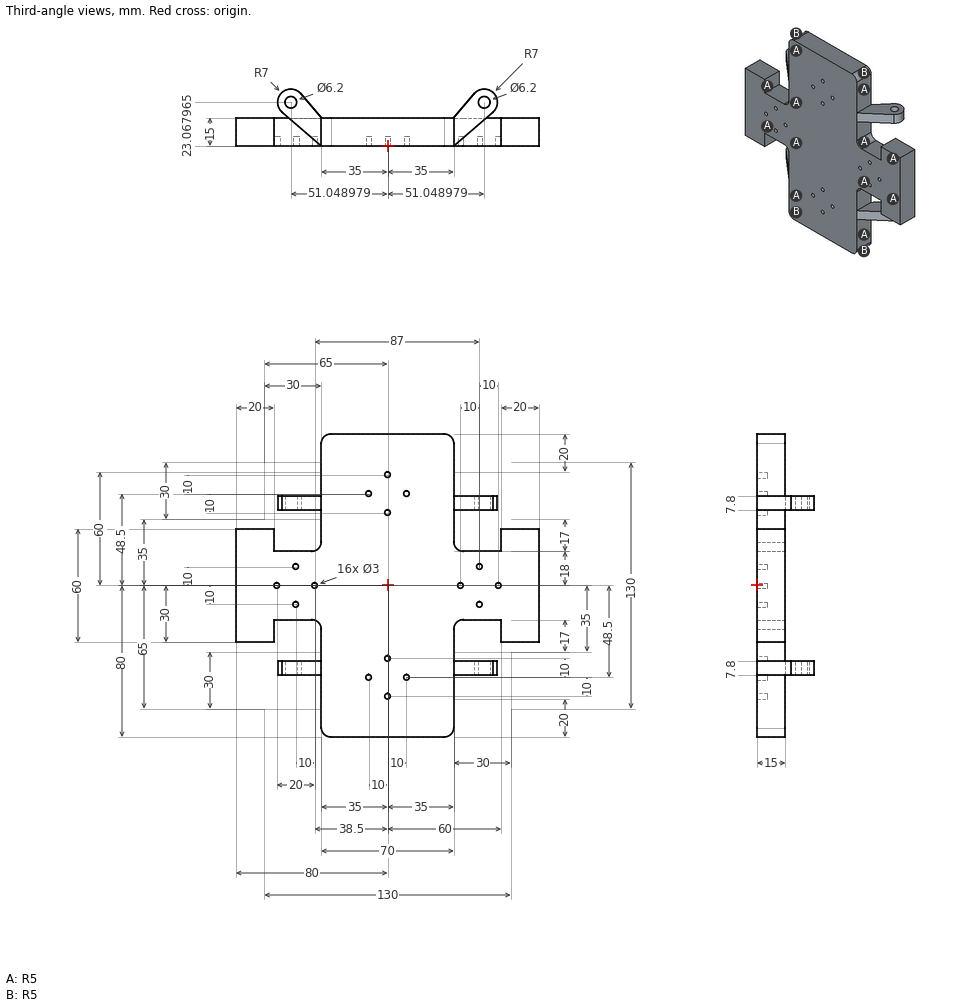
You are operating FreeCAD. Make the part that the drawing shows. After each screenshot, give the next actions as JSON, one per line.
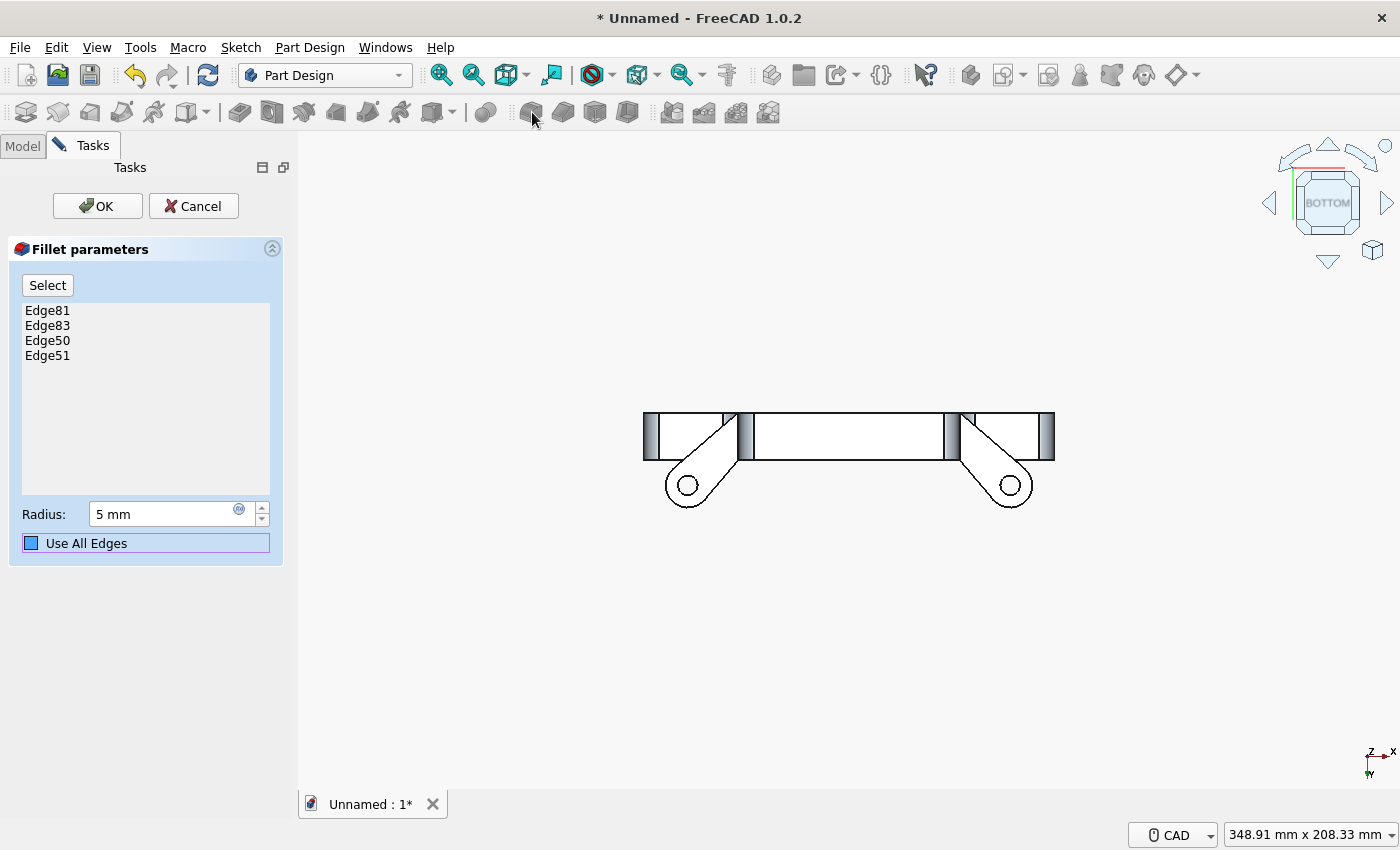
{"action": "left_click", "coordinate": [98, 206]}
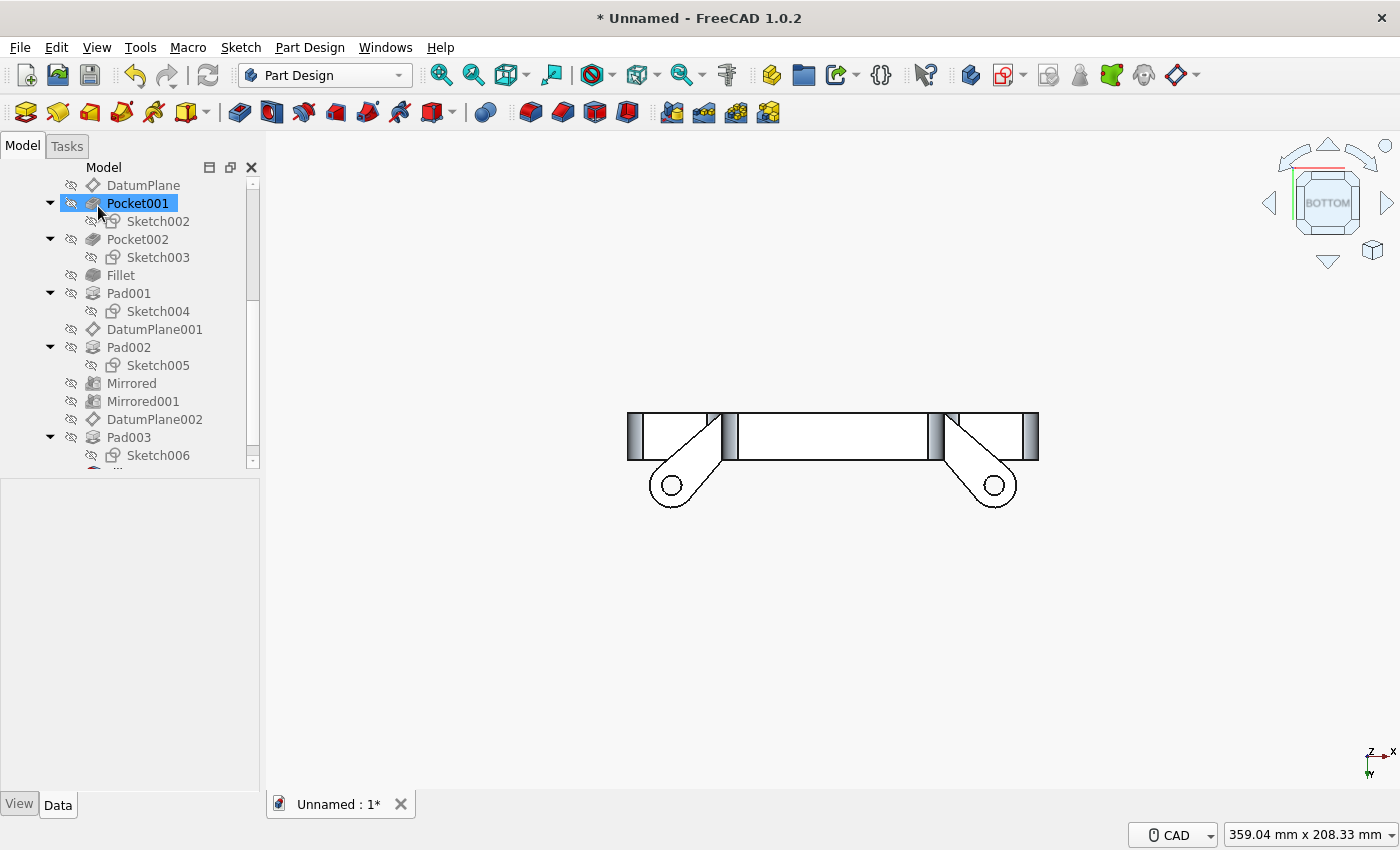
{"action": "left_click", "coordinate": [442, 76]}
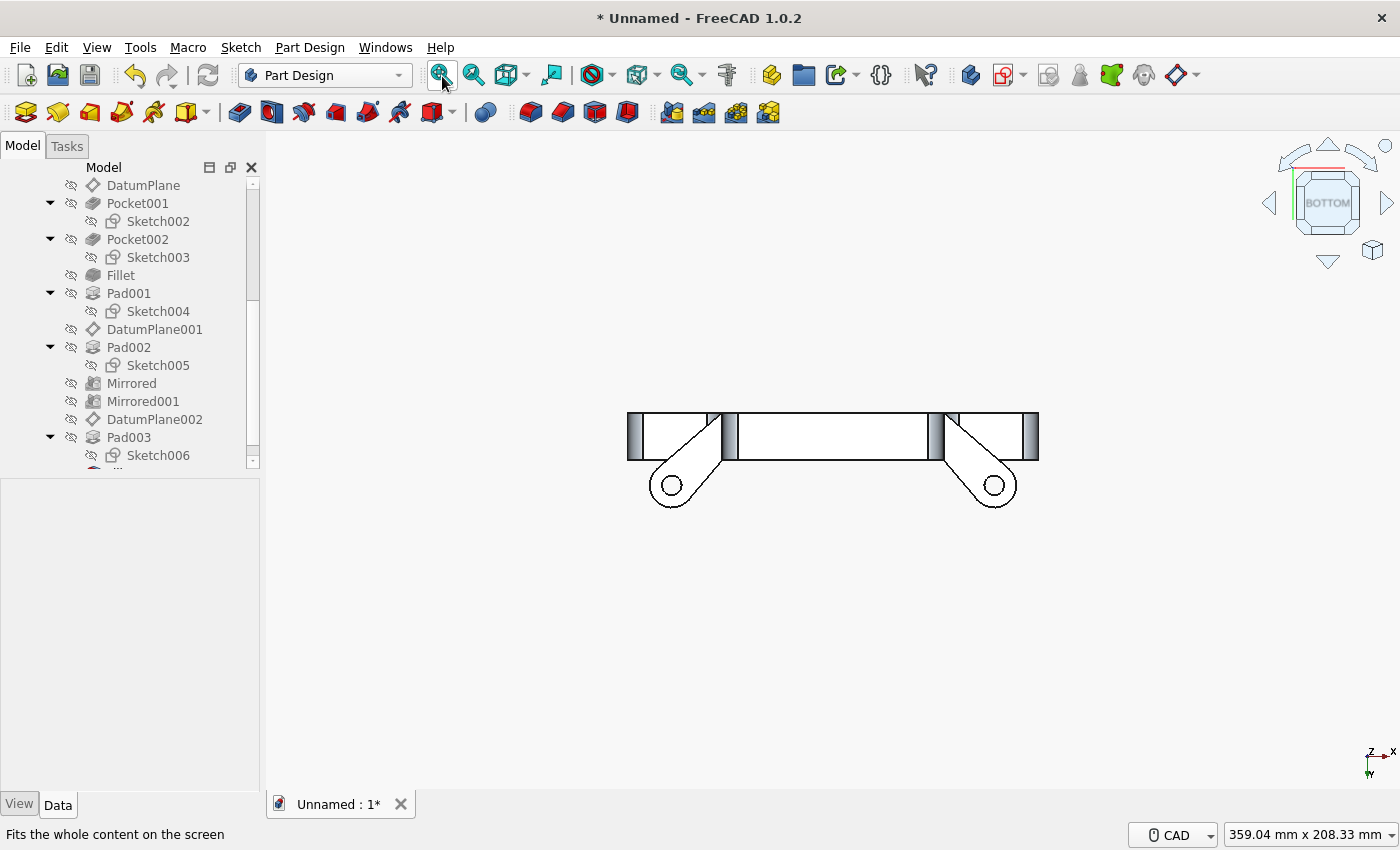
{"action": "key", "text": "4"}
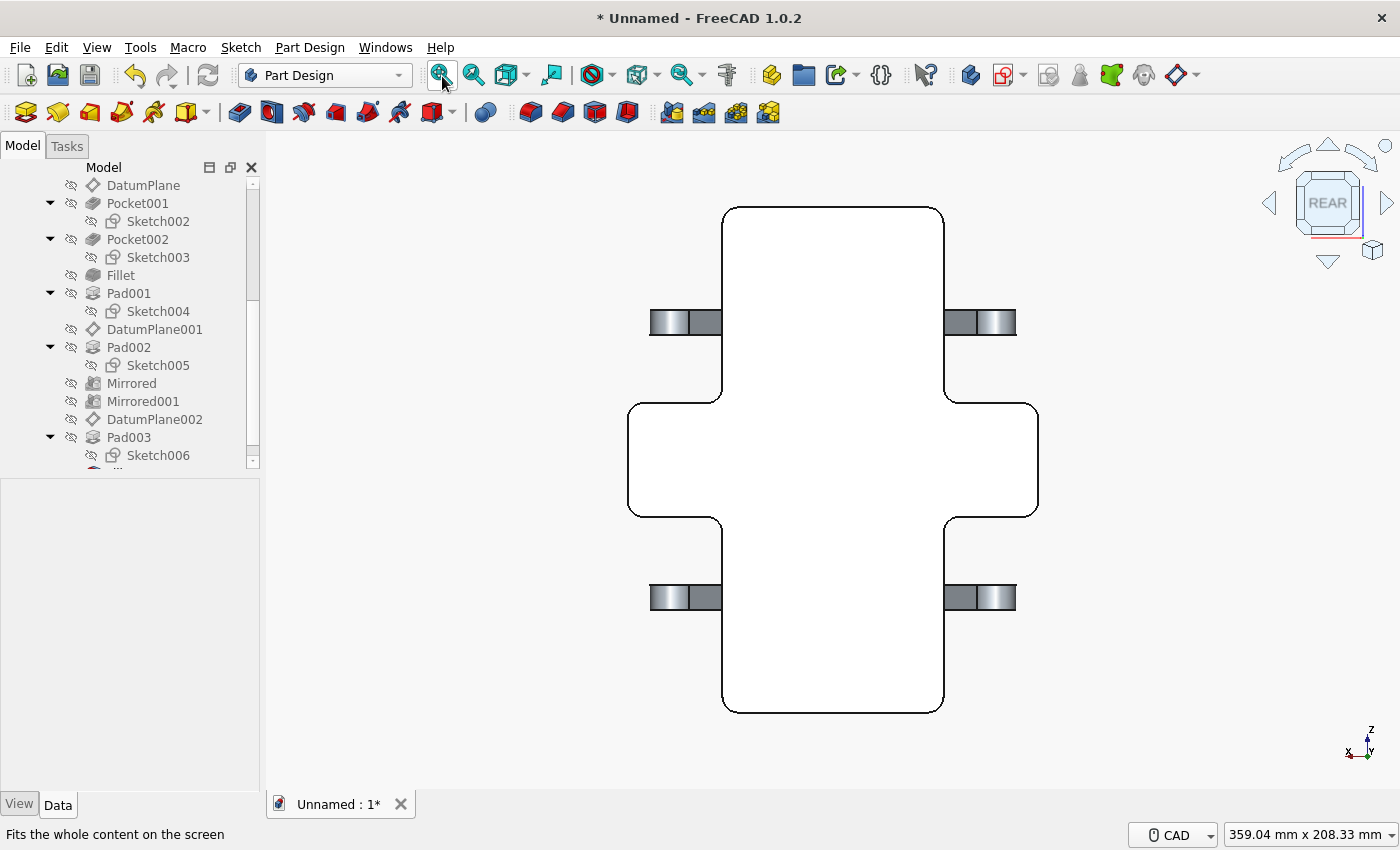
{"action": "left_click", "coordinate": [833, 459]}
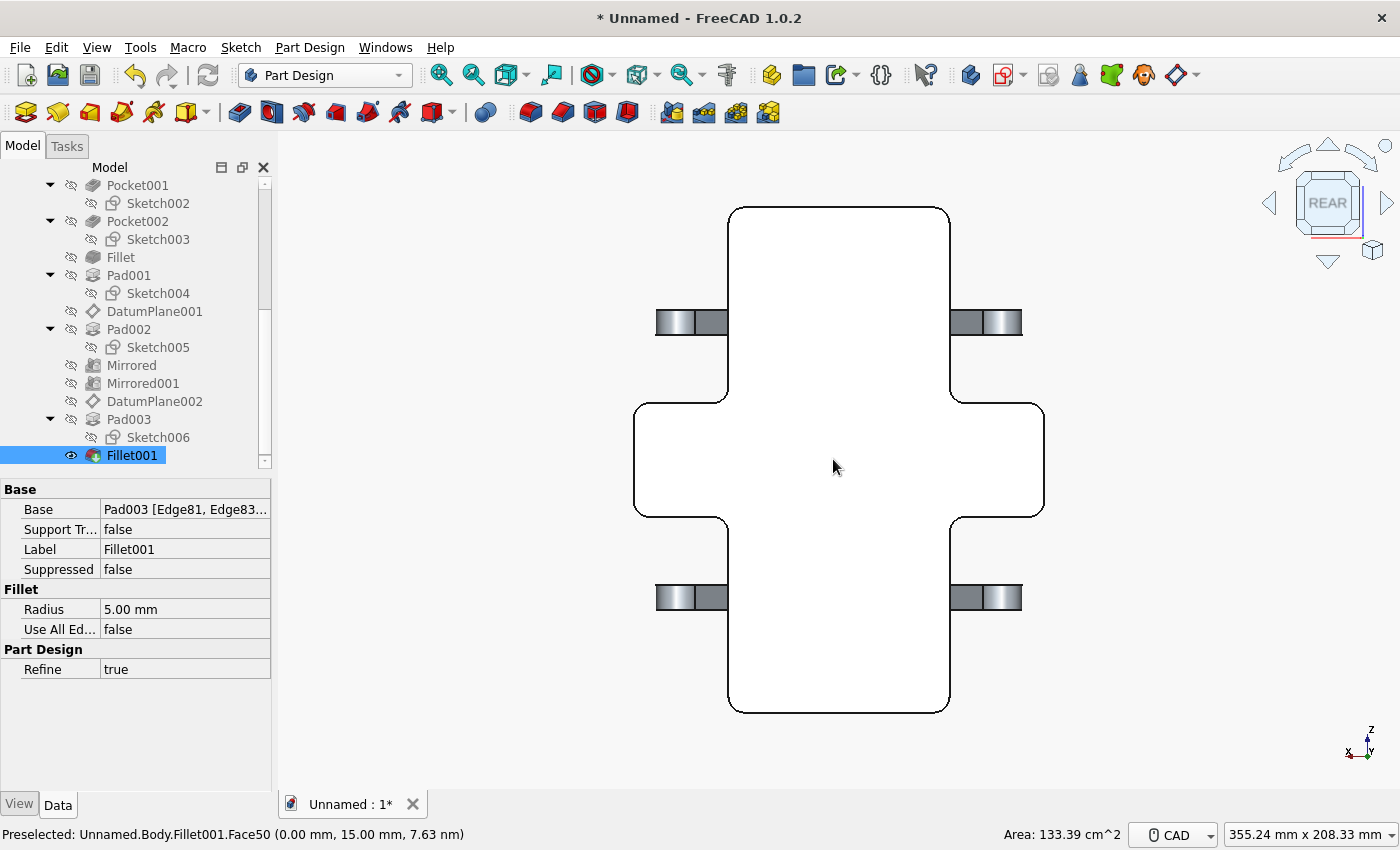
{"action": "left_click", "coordinate": [1004, 76]}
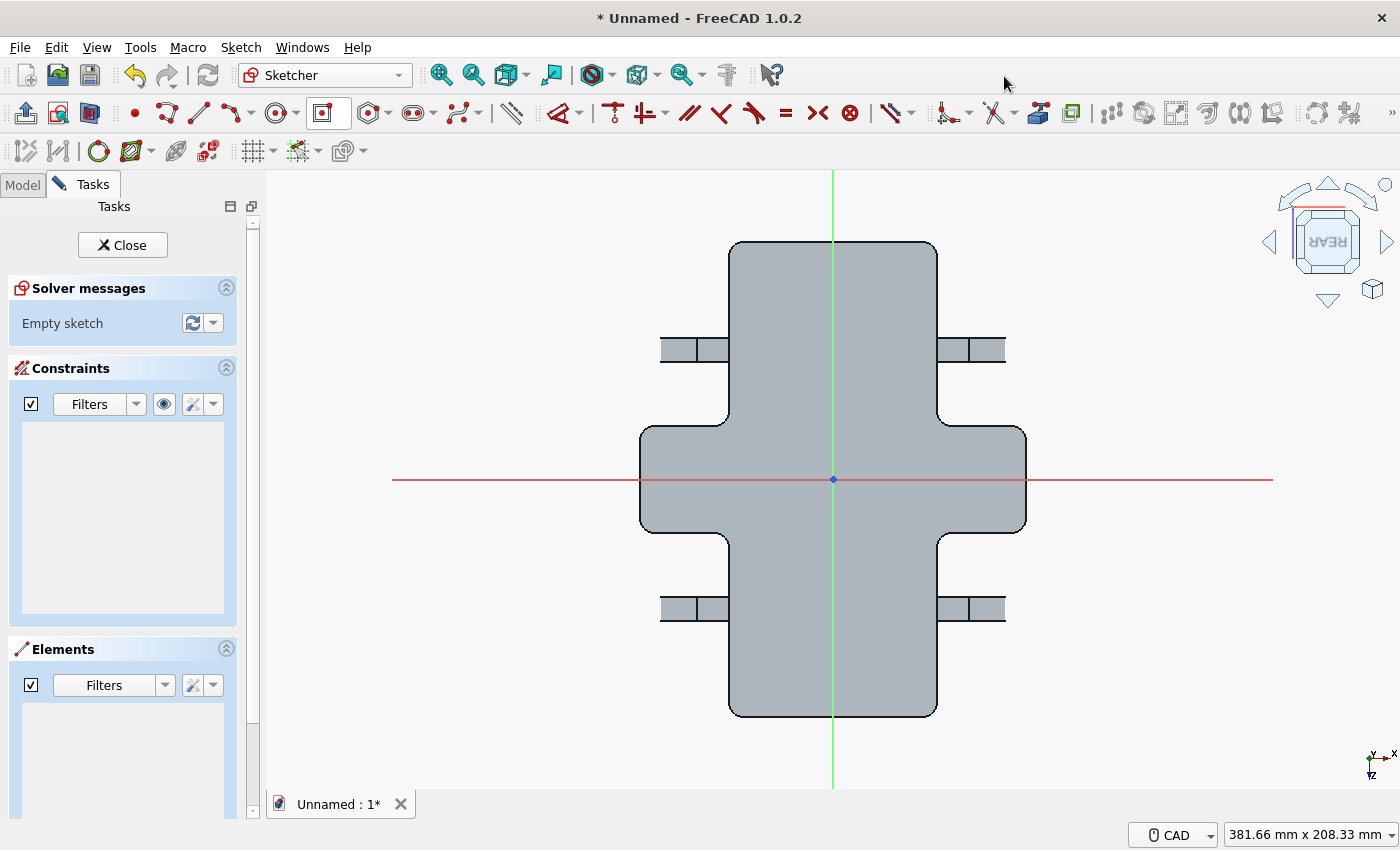
{"action": "scroll", "coordinate": [972, 479], "scroll_direction": "up", "scroll_amount": 2}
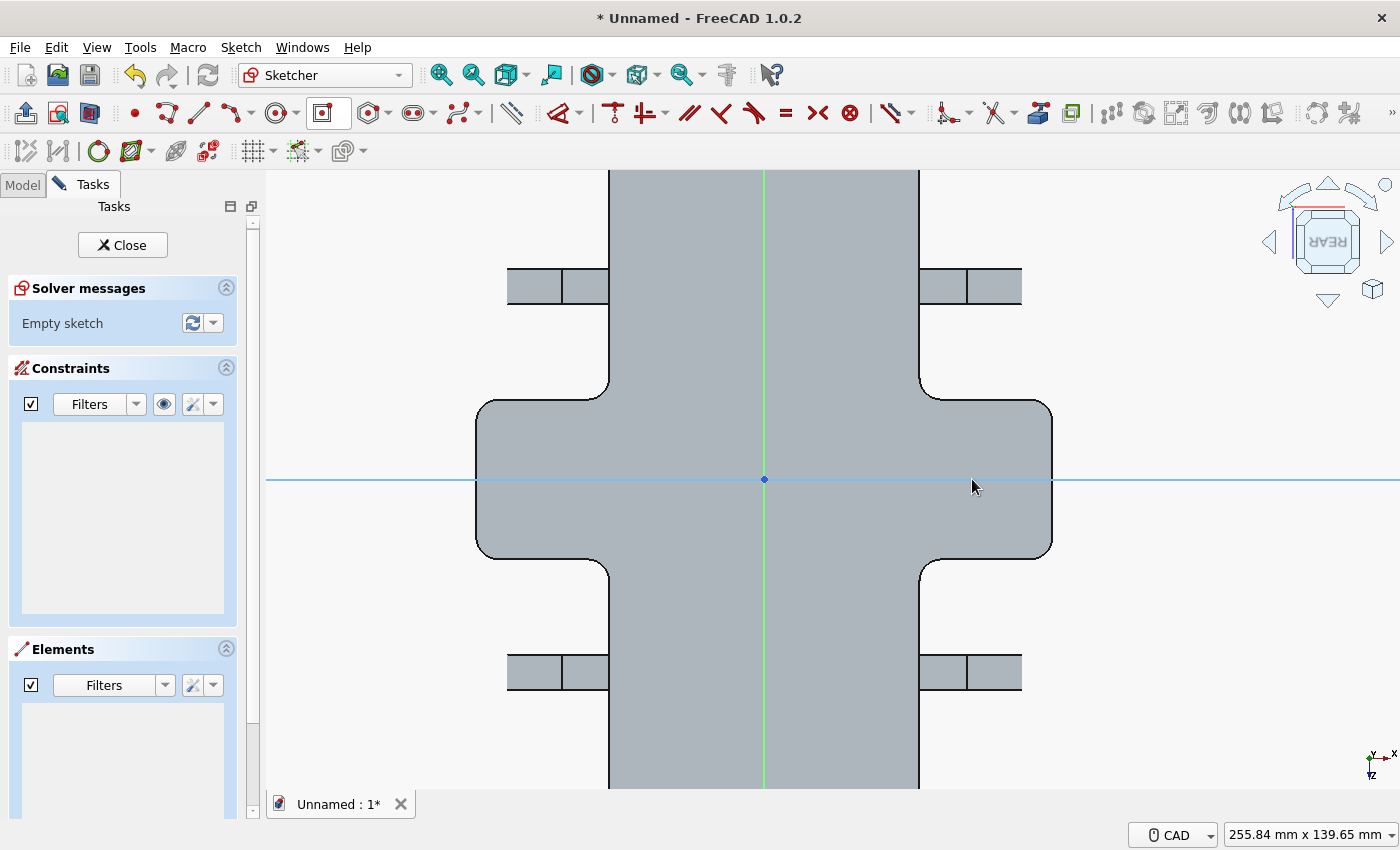
{"action": "key", "text": "g r"}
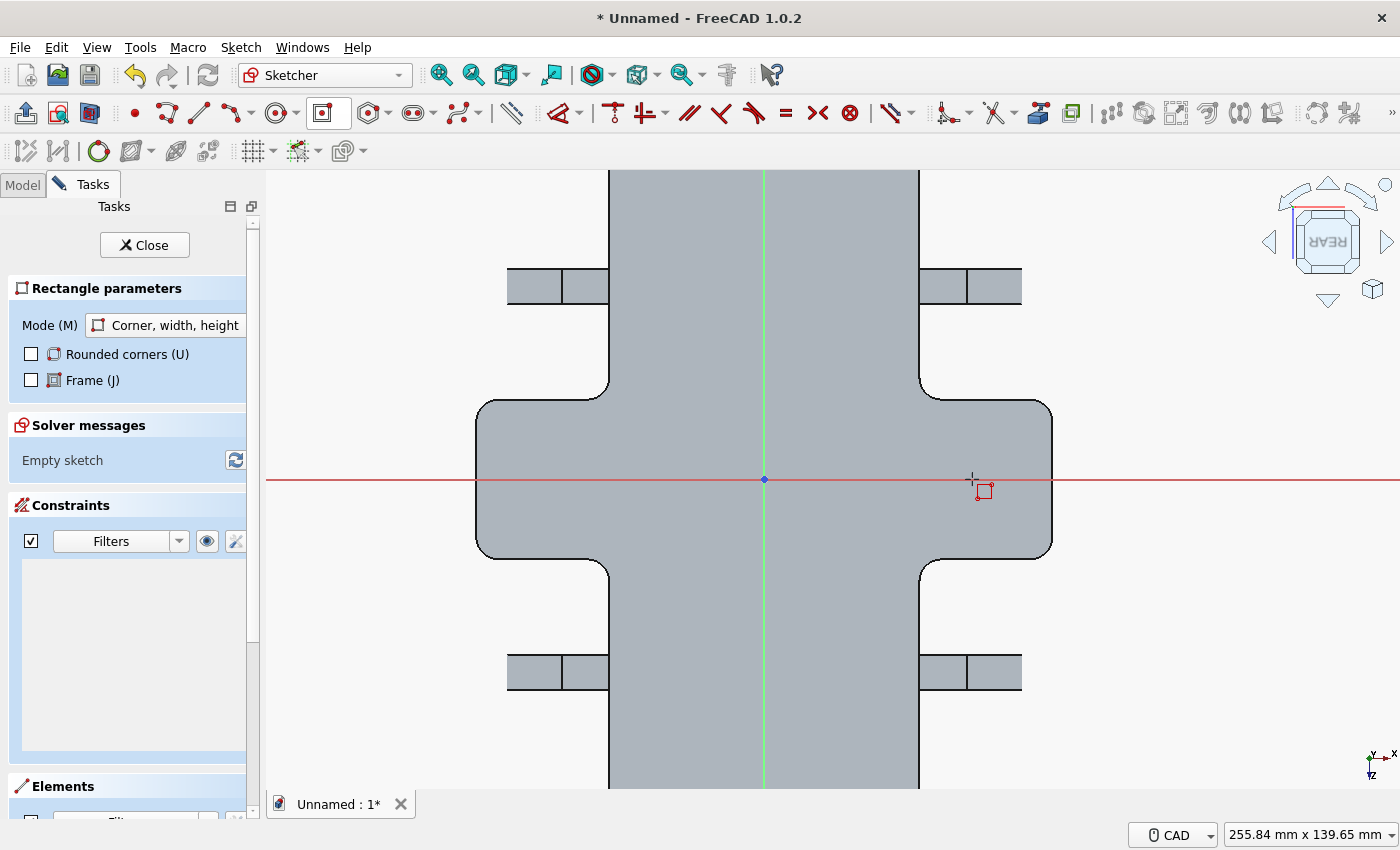
{"action": "left_click", "coordinate": [410, 347]}
{"action": "mouse_move", "coordinate": [498, 612]}